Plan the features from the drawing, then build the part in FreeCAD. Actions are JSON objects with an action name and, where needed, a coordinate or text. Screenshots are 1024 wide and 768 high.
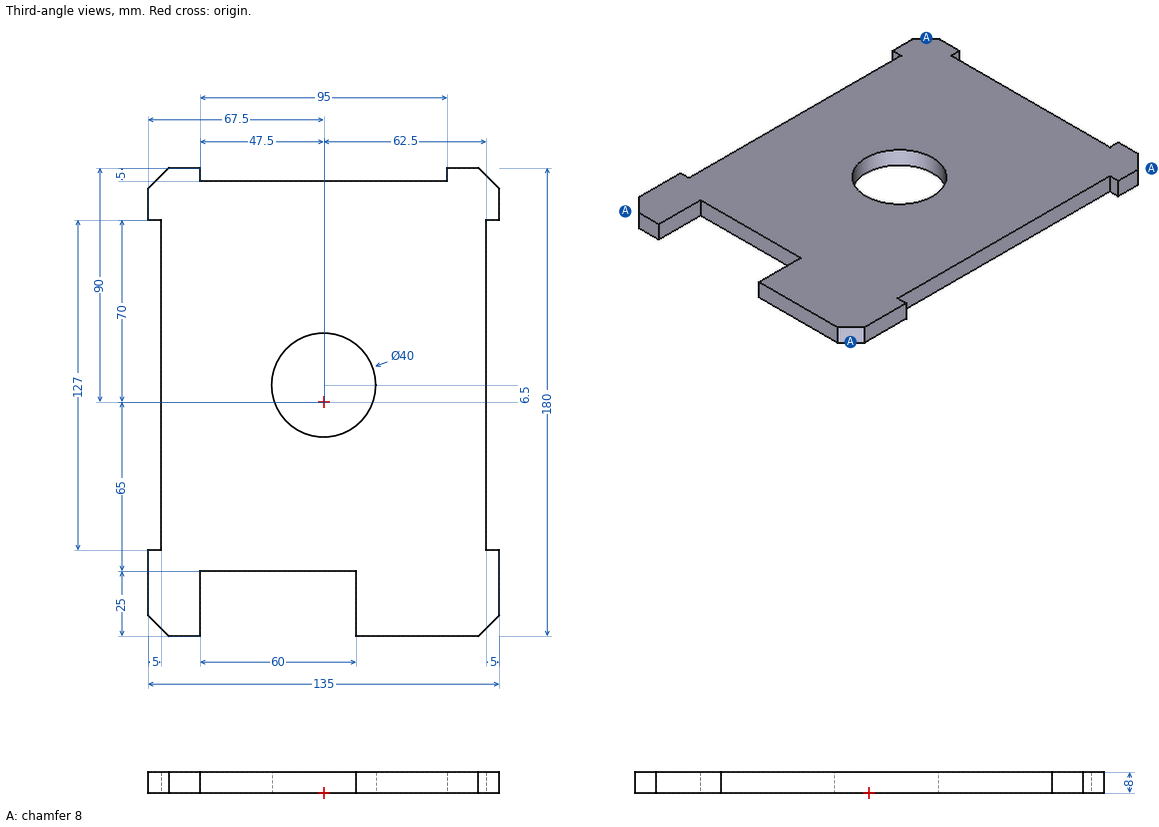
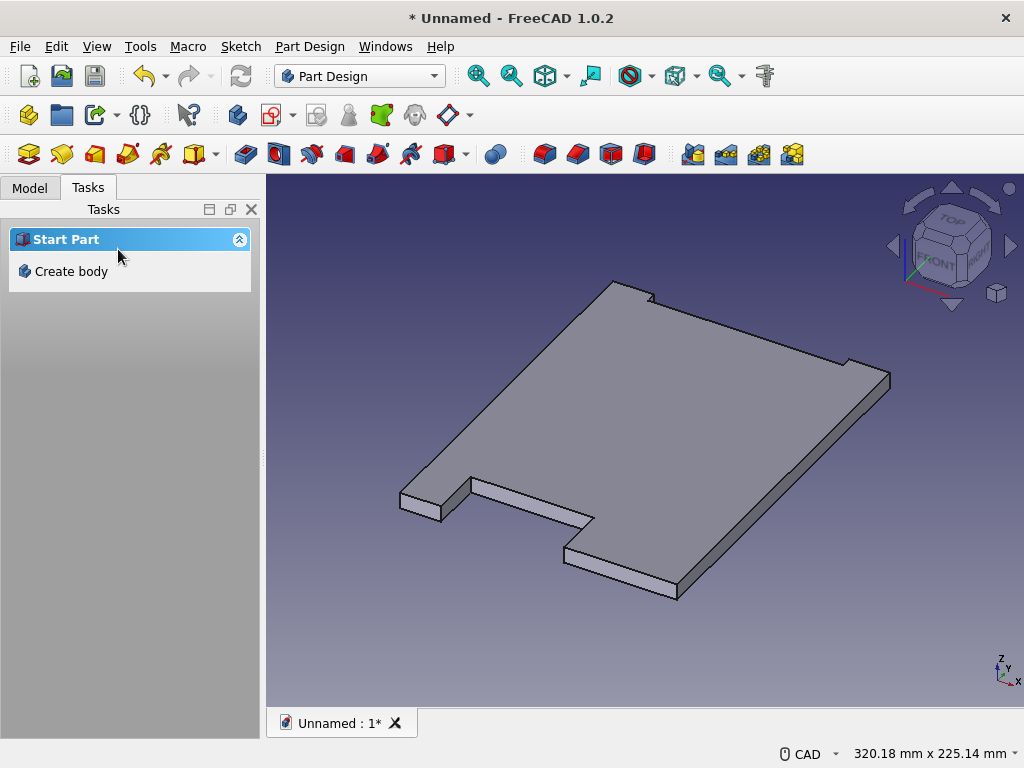
{"action": "left_click", "coordinate": [645, 432]}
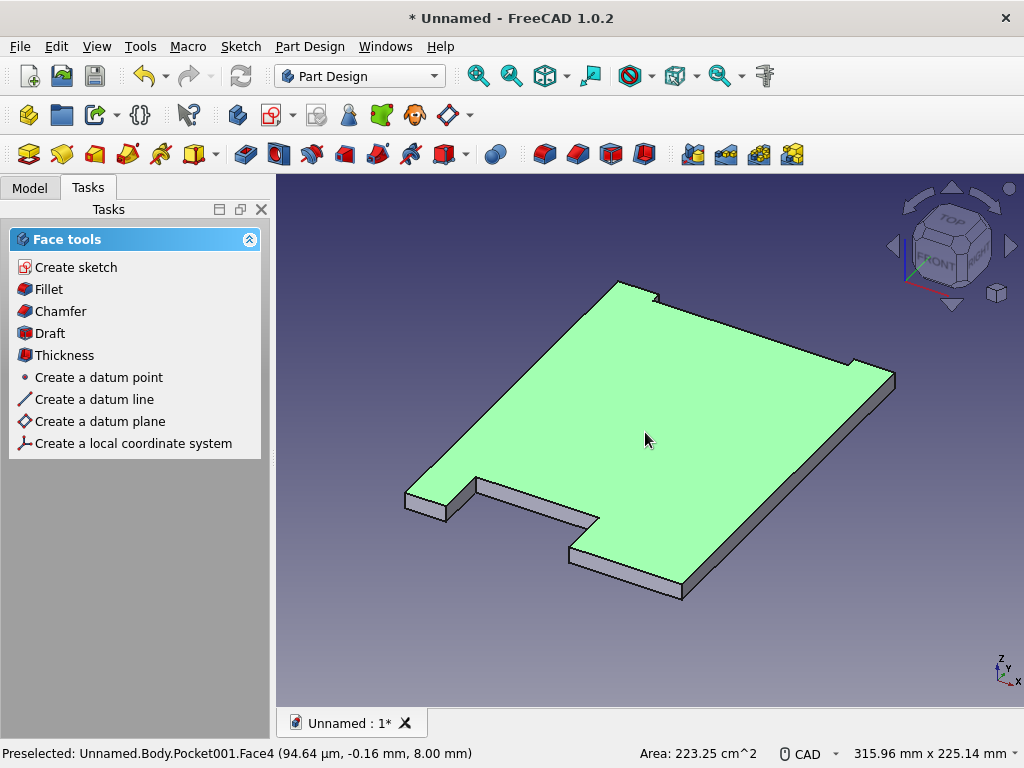
{"action": "left_click", "coordinate": [270, 116]}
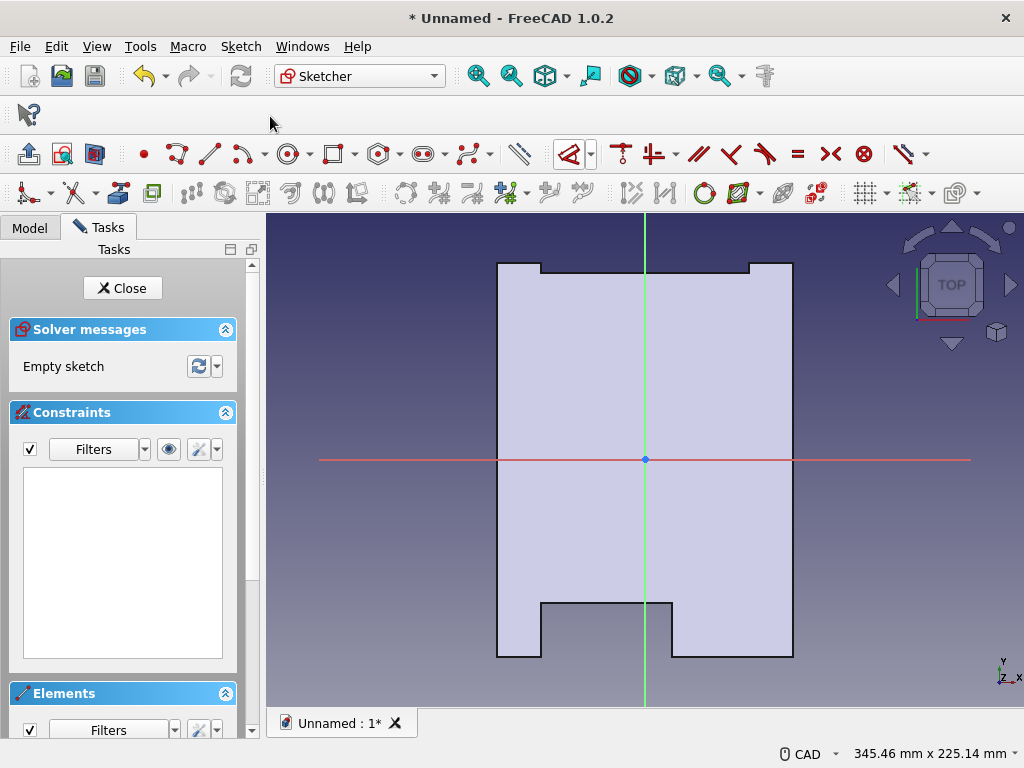
{"action": "key", "text": "g r"}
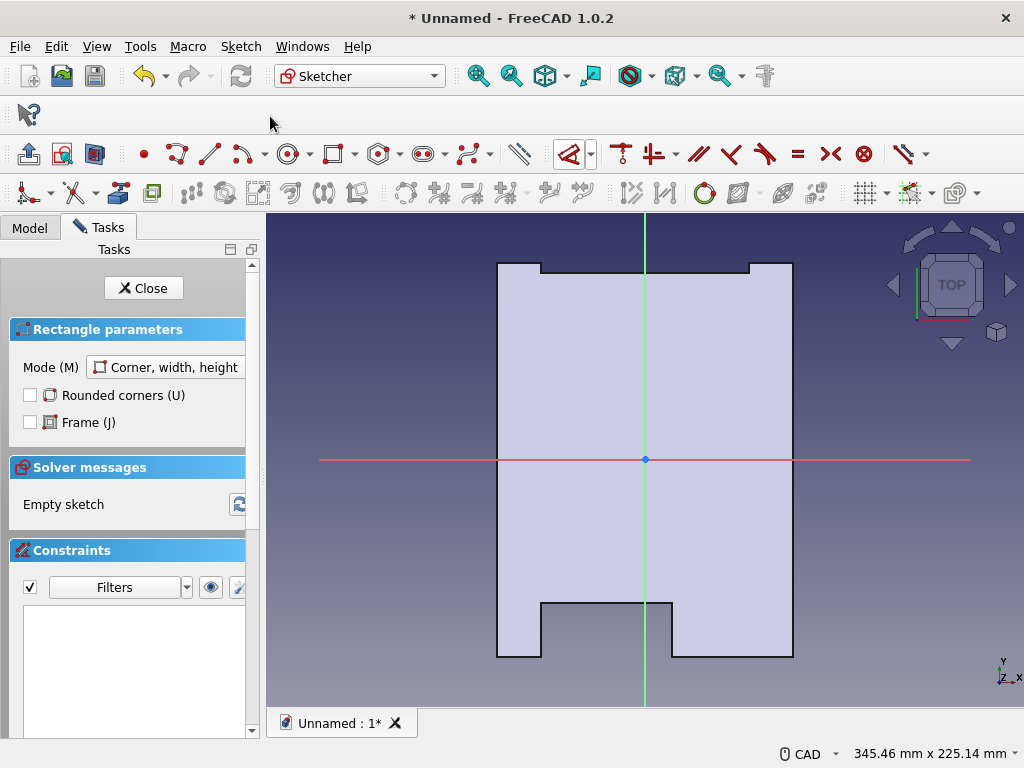
{"action": "scroll", "coordinate": [497, 306], "scroll_direction": "up", "scroll_amount": 2}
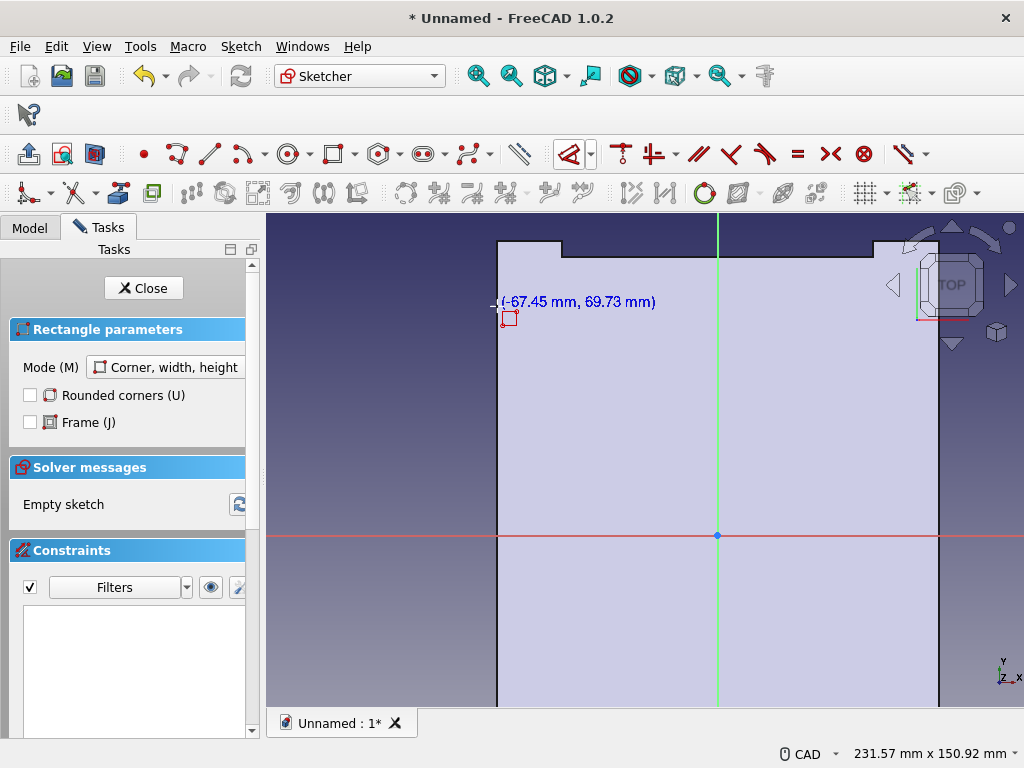
{"action": "left_click", "coordinate": [497, 307]}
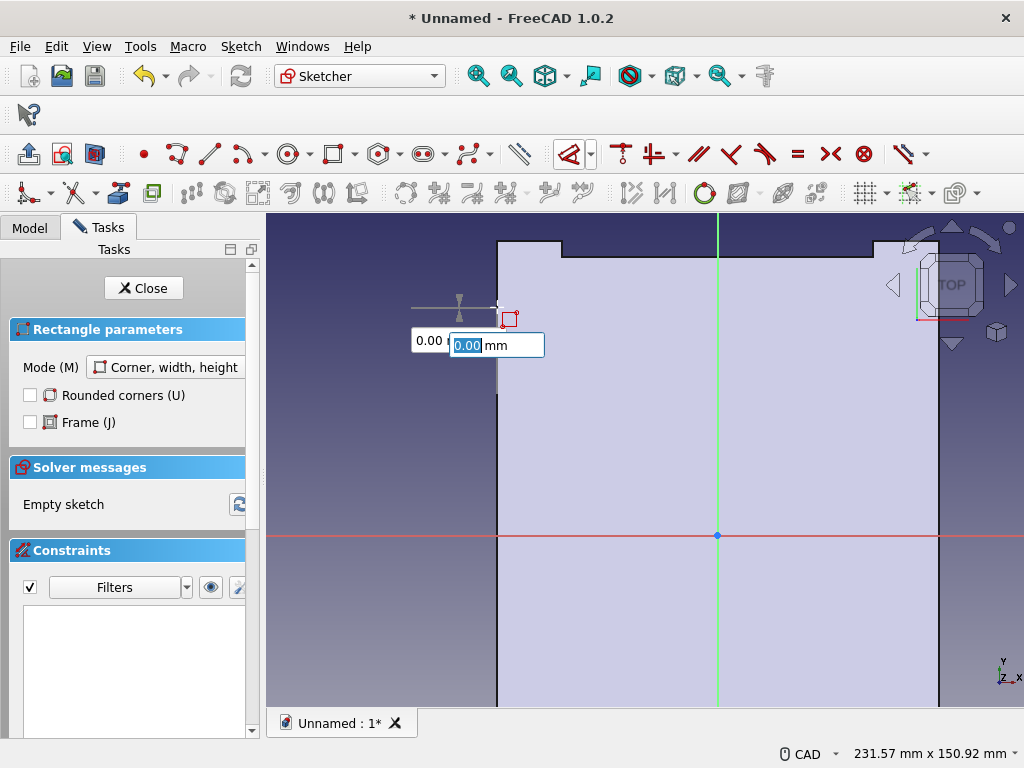
{"action": "scroll", "coordinate": [438, 241], "scroll_direction": "down", "scroll_amount": 1}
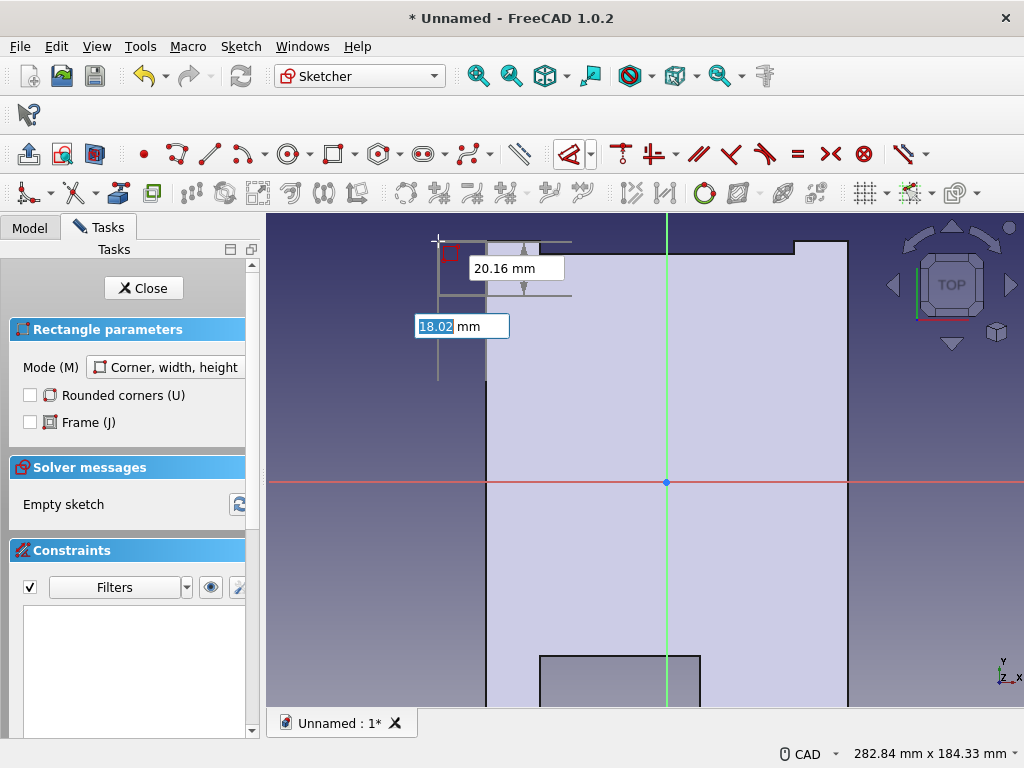
{"action": "left_click", "coordinate": [499, 635]}
{"action": "key", "text": "Escape"}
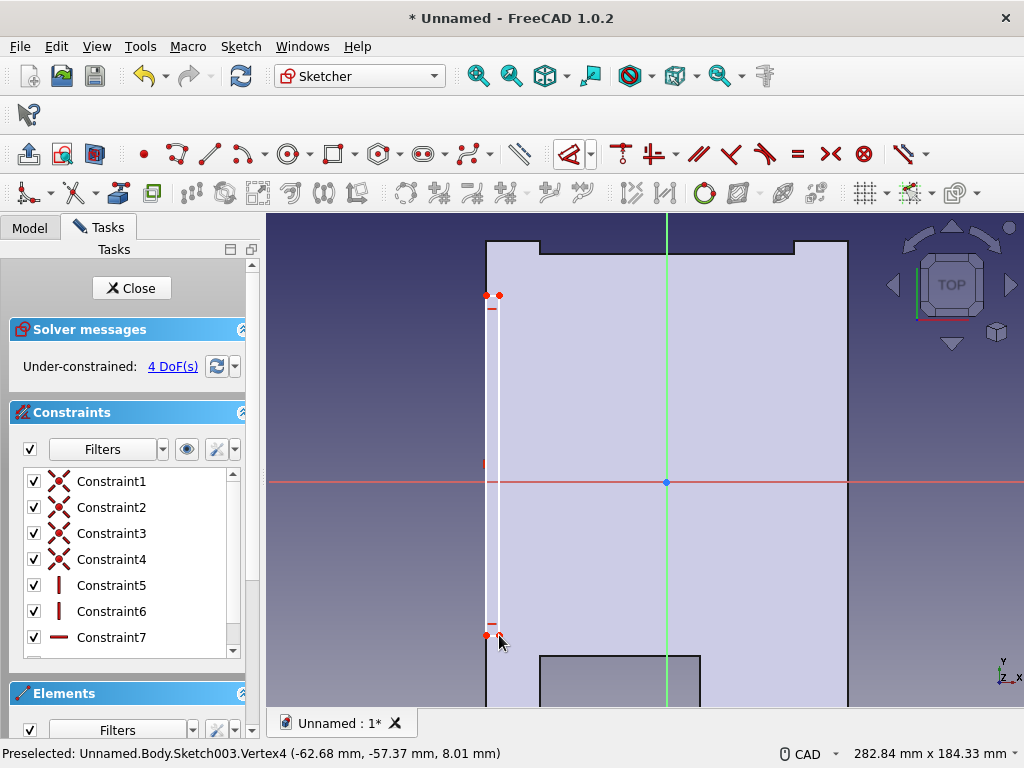
{"action": "scroll", "coordinate": [493, 636], "scroll_direction": "up", "scroll_amount": 6}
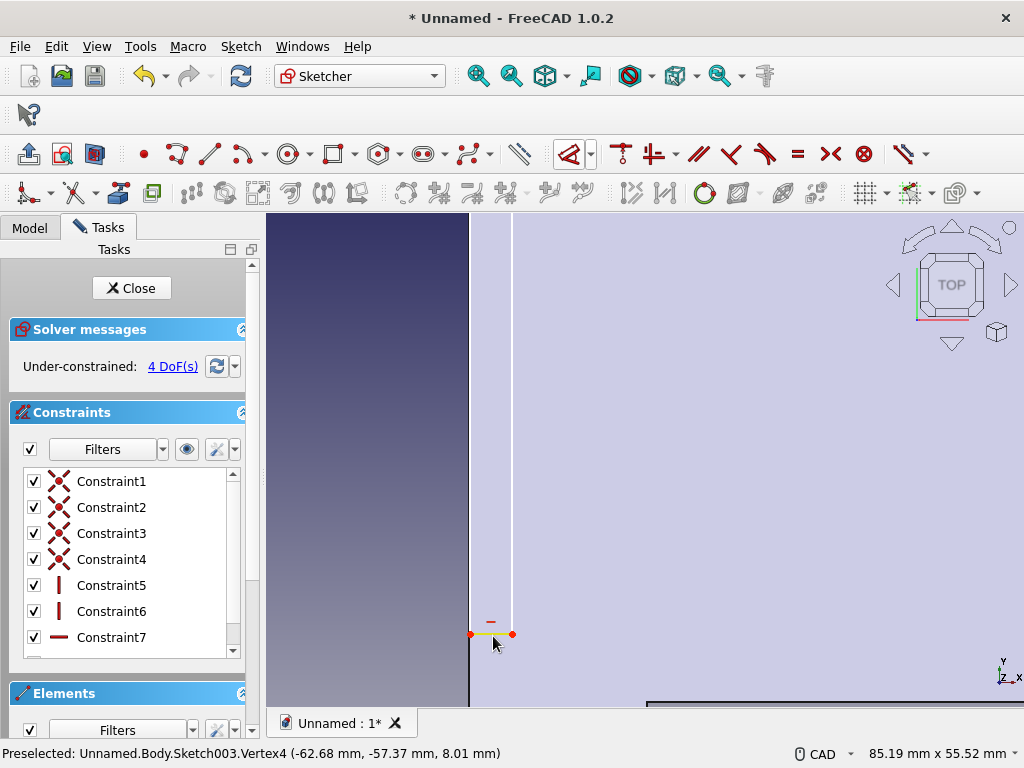
{"action": "left_click", "coordinate": [491, 634]}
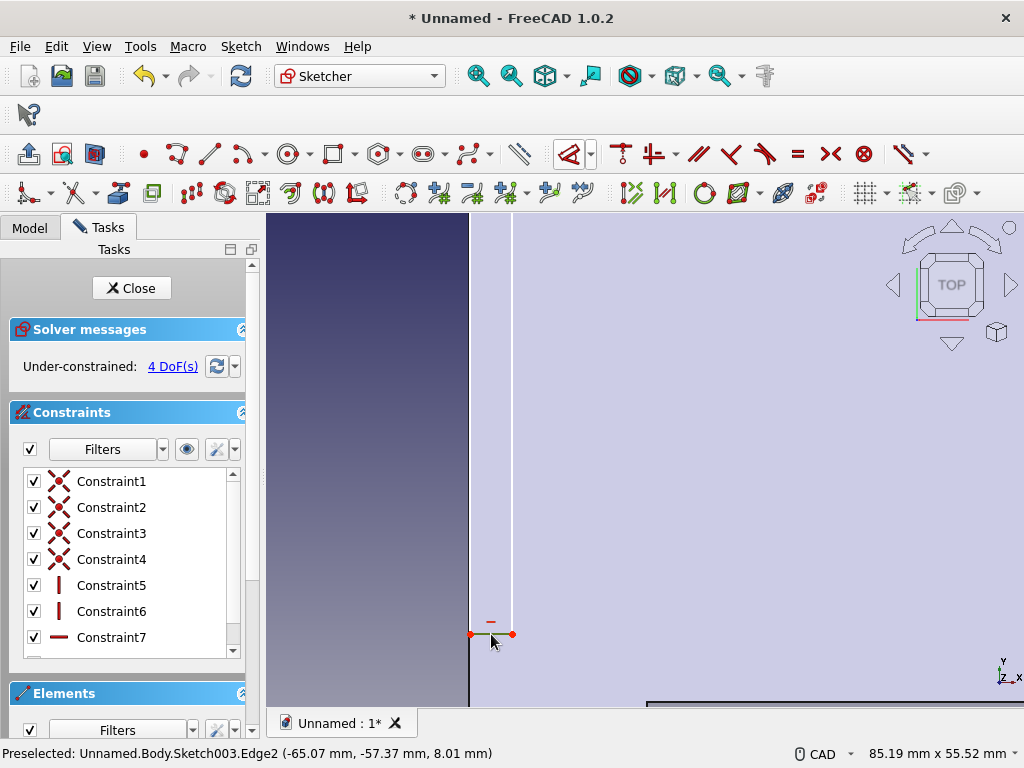
{"action": "left_click", "coordinate": [590, 154]}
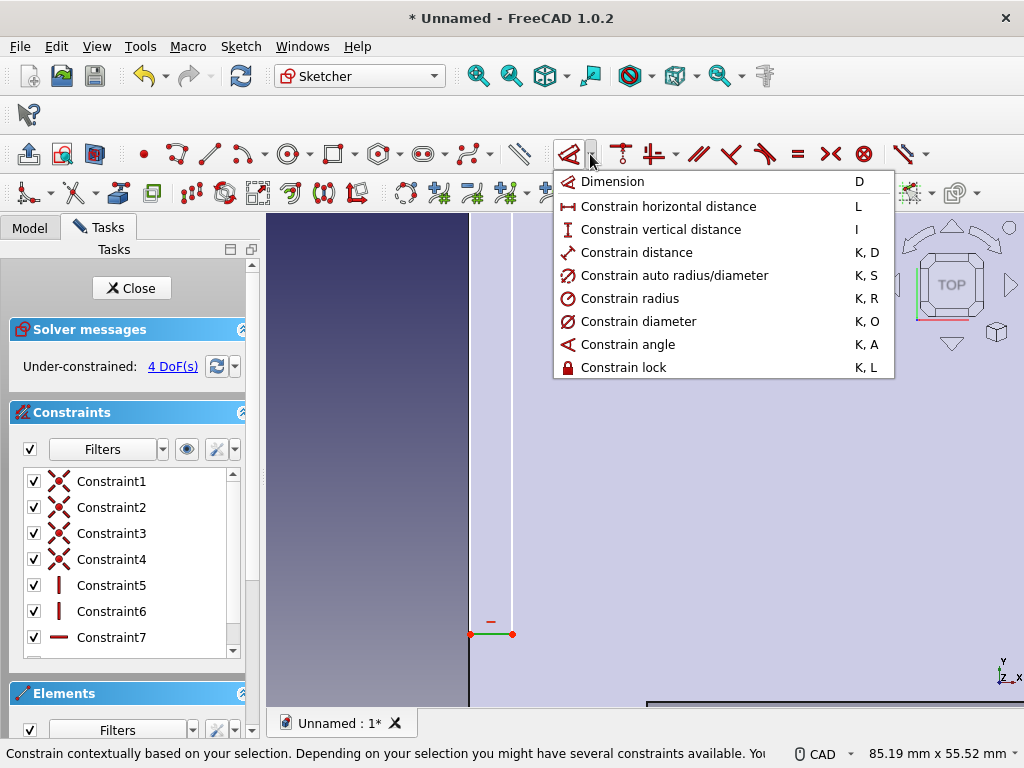
{"action": "left_click", "coordinate": [724, 206]}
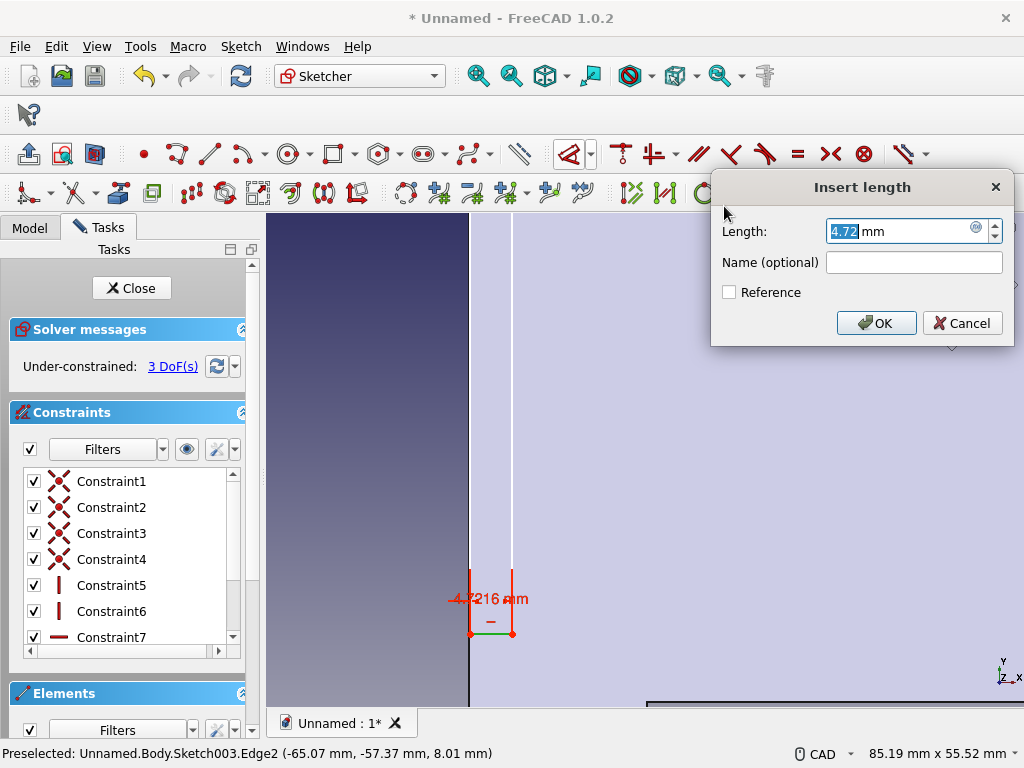
{"action": "type", "text": "5"}
{"action": "key", "text": "Return"}